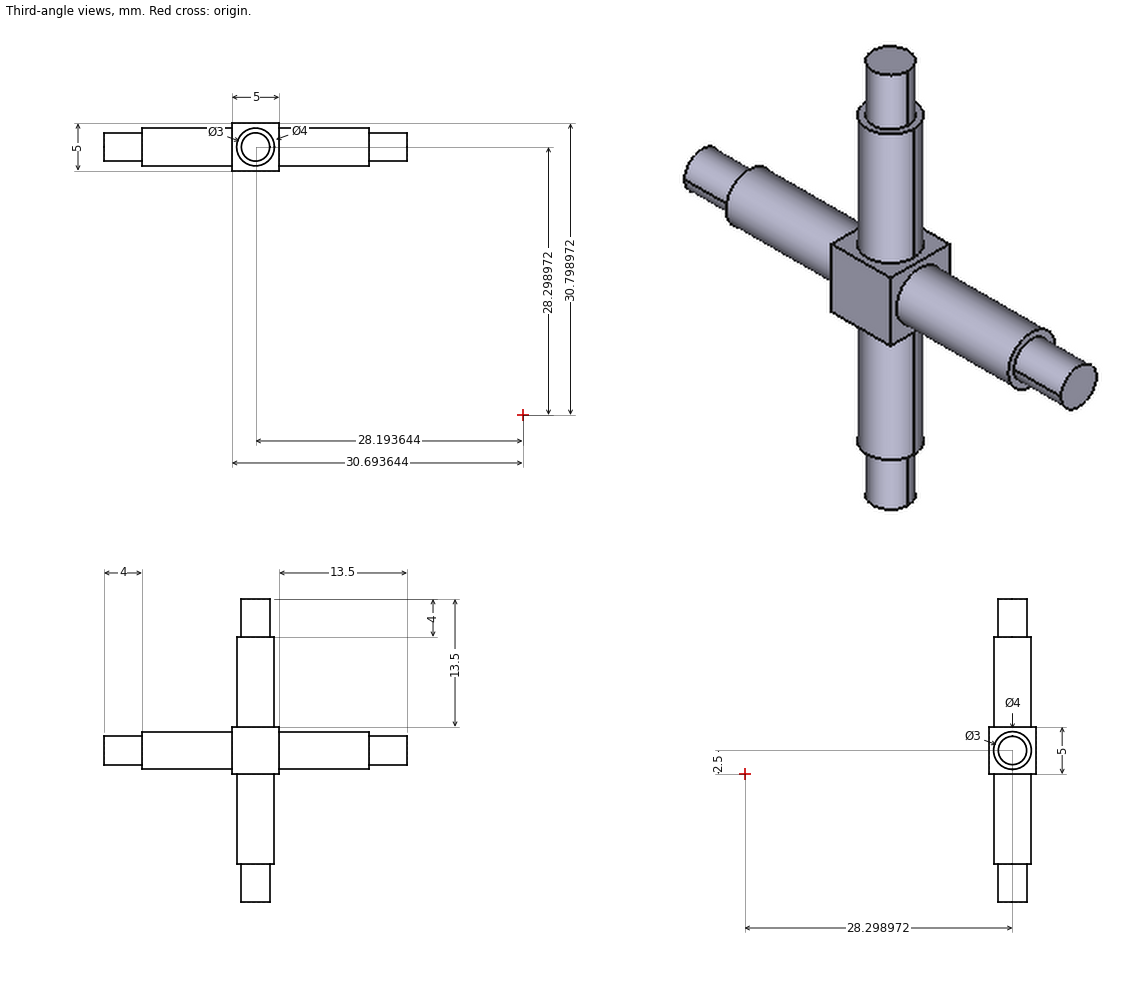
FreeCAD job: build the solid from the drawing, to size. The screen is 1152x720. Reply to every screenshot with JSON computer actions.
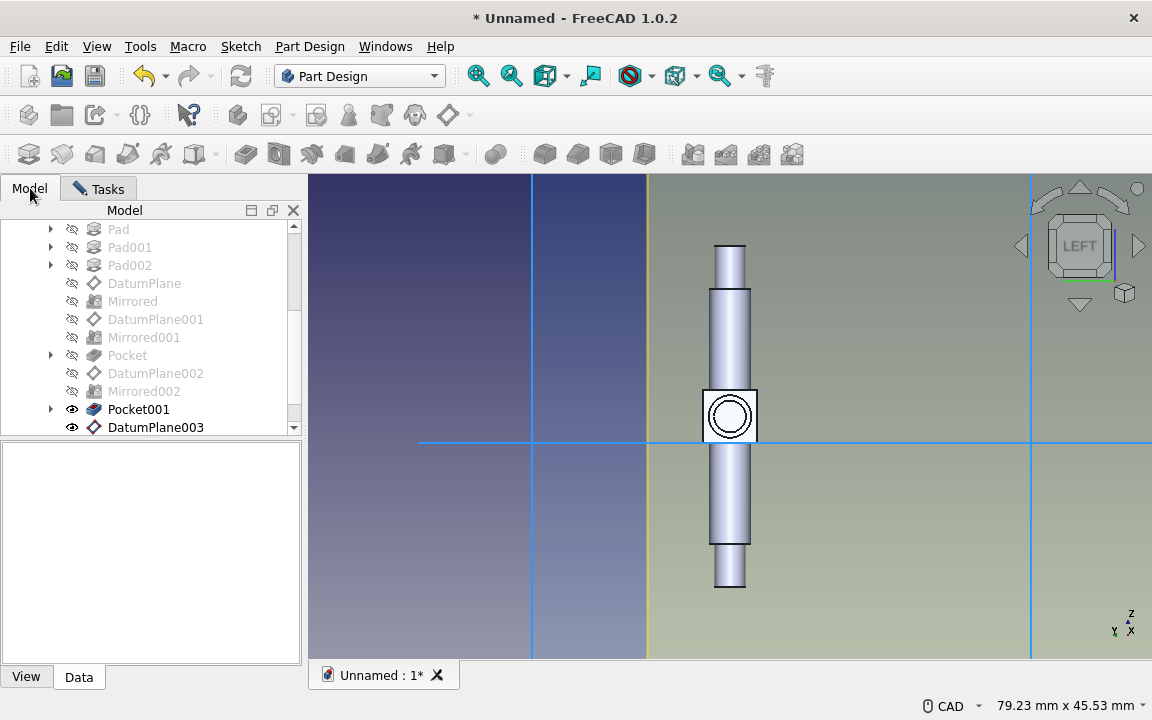
{"action": "left_click", "coordinate": [117, 427]}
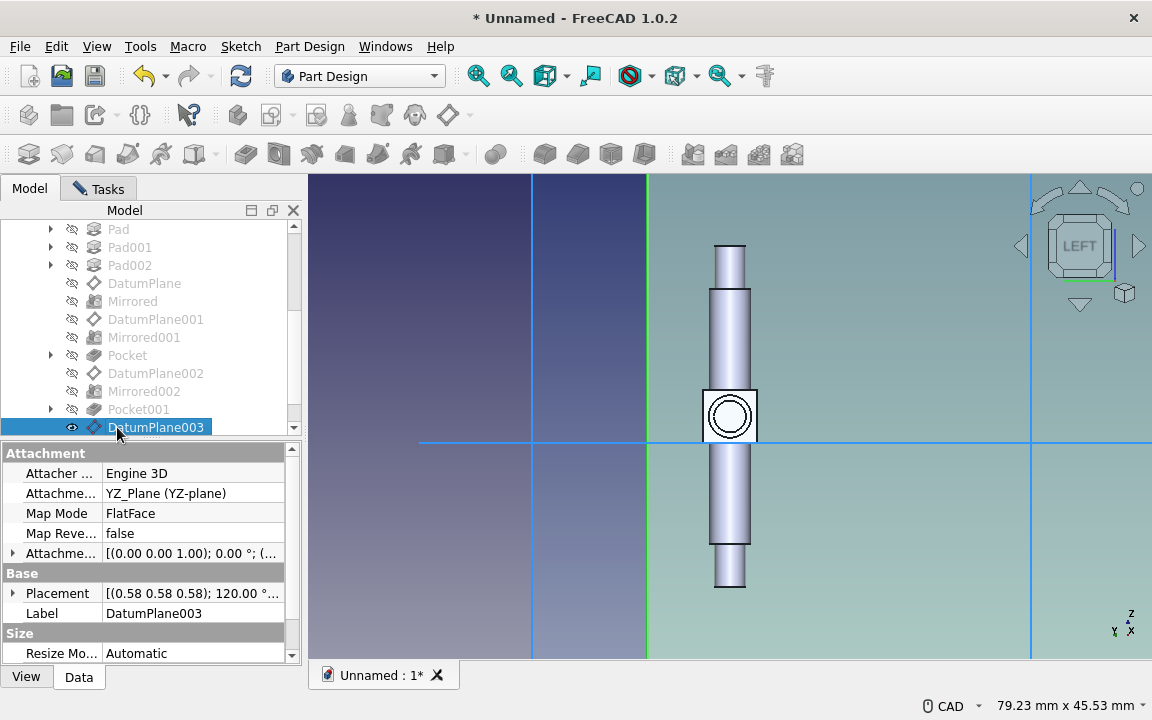
{"action": "left_click", "coordinate": [98, 188]}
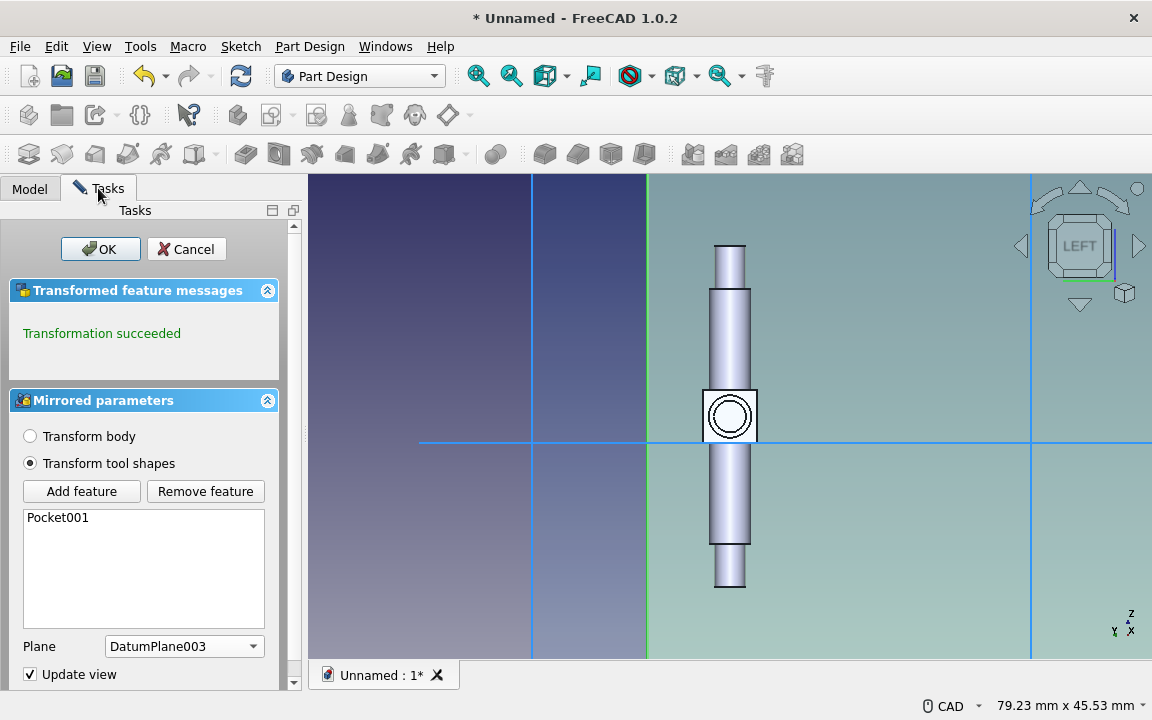
{"action": "left_click", "coordinate": [101, 249]}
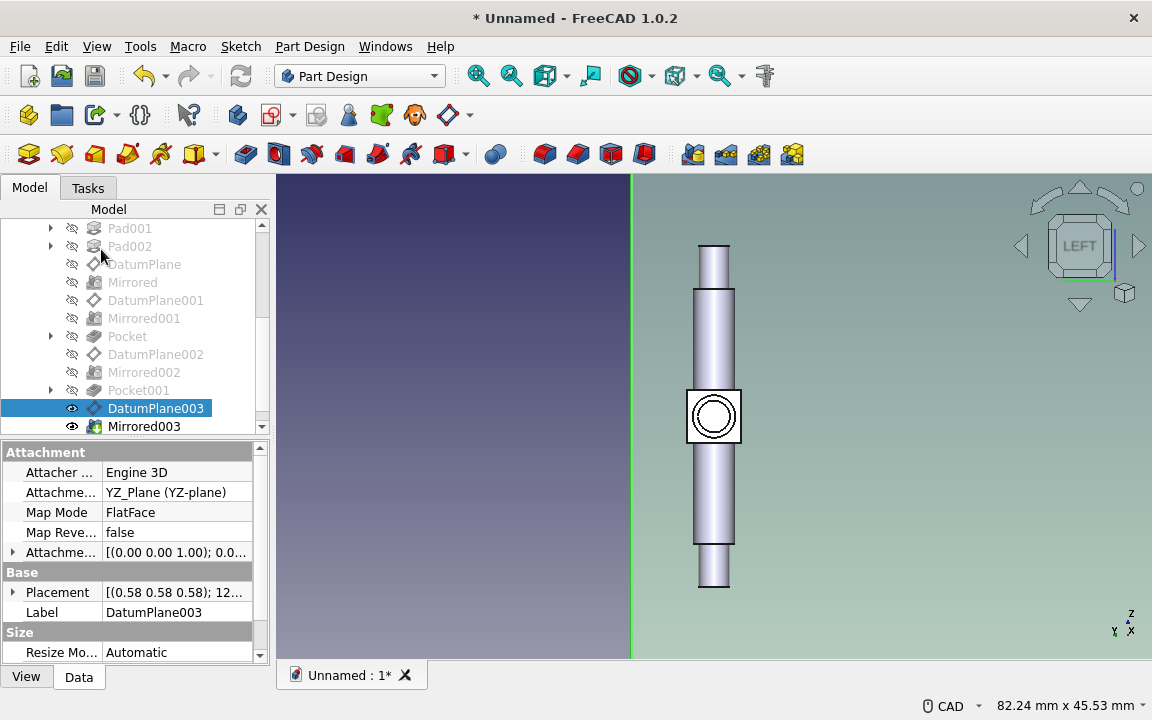
{"action": "left_click", "coordinate": [117, 408]}
{"action": "key", "text": "space"}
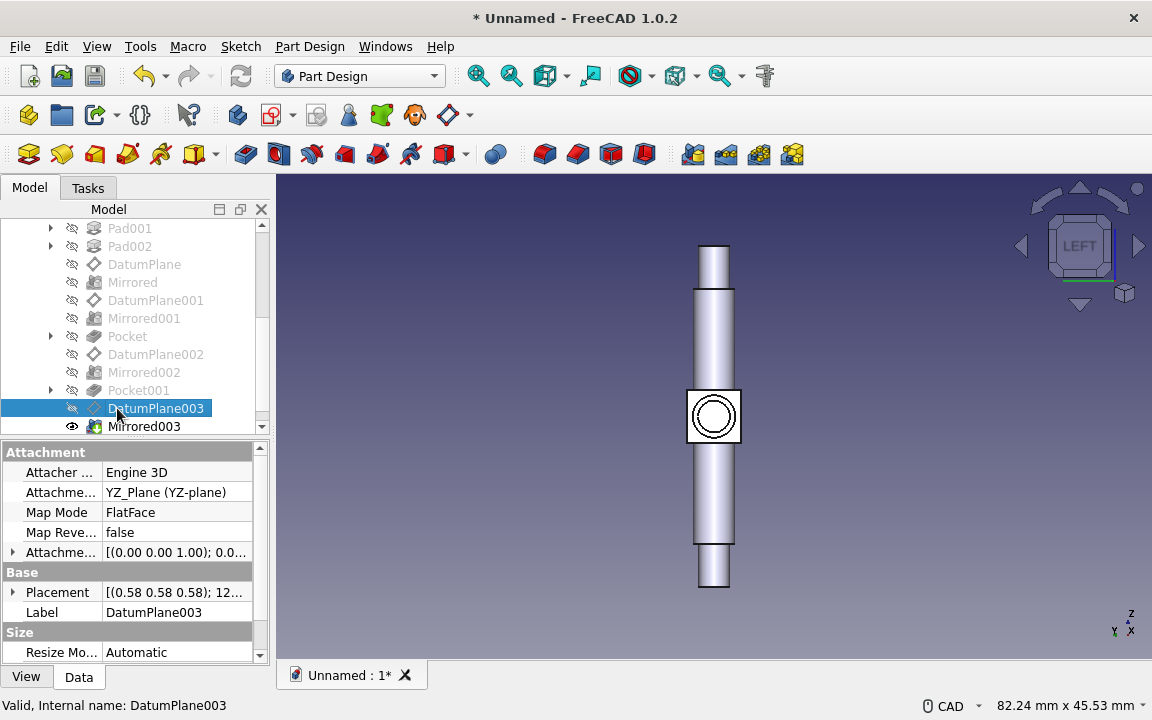
{"action": "key", "text": "0"}